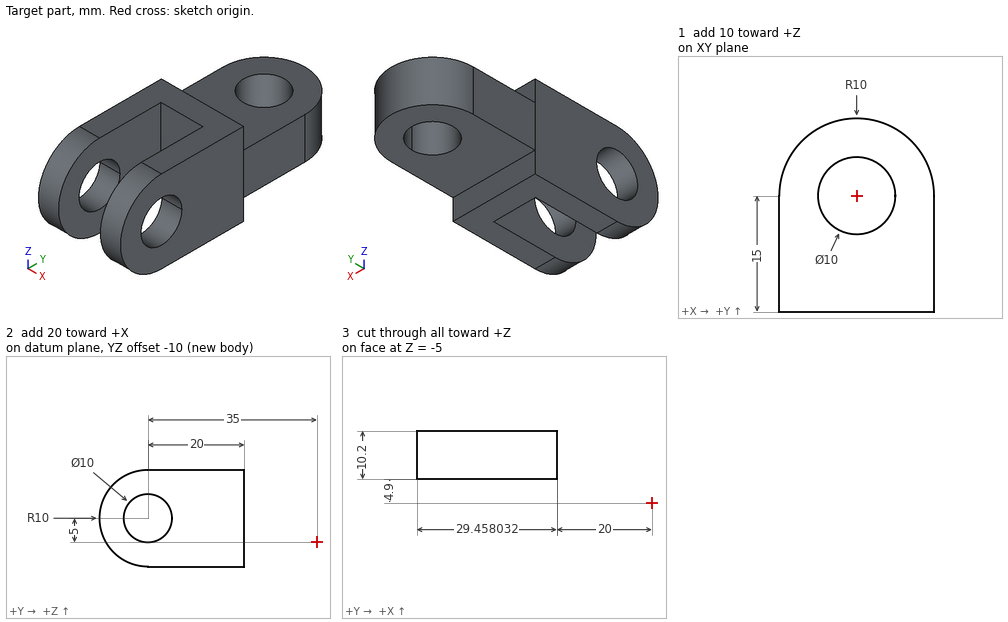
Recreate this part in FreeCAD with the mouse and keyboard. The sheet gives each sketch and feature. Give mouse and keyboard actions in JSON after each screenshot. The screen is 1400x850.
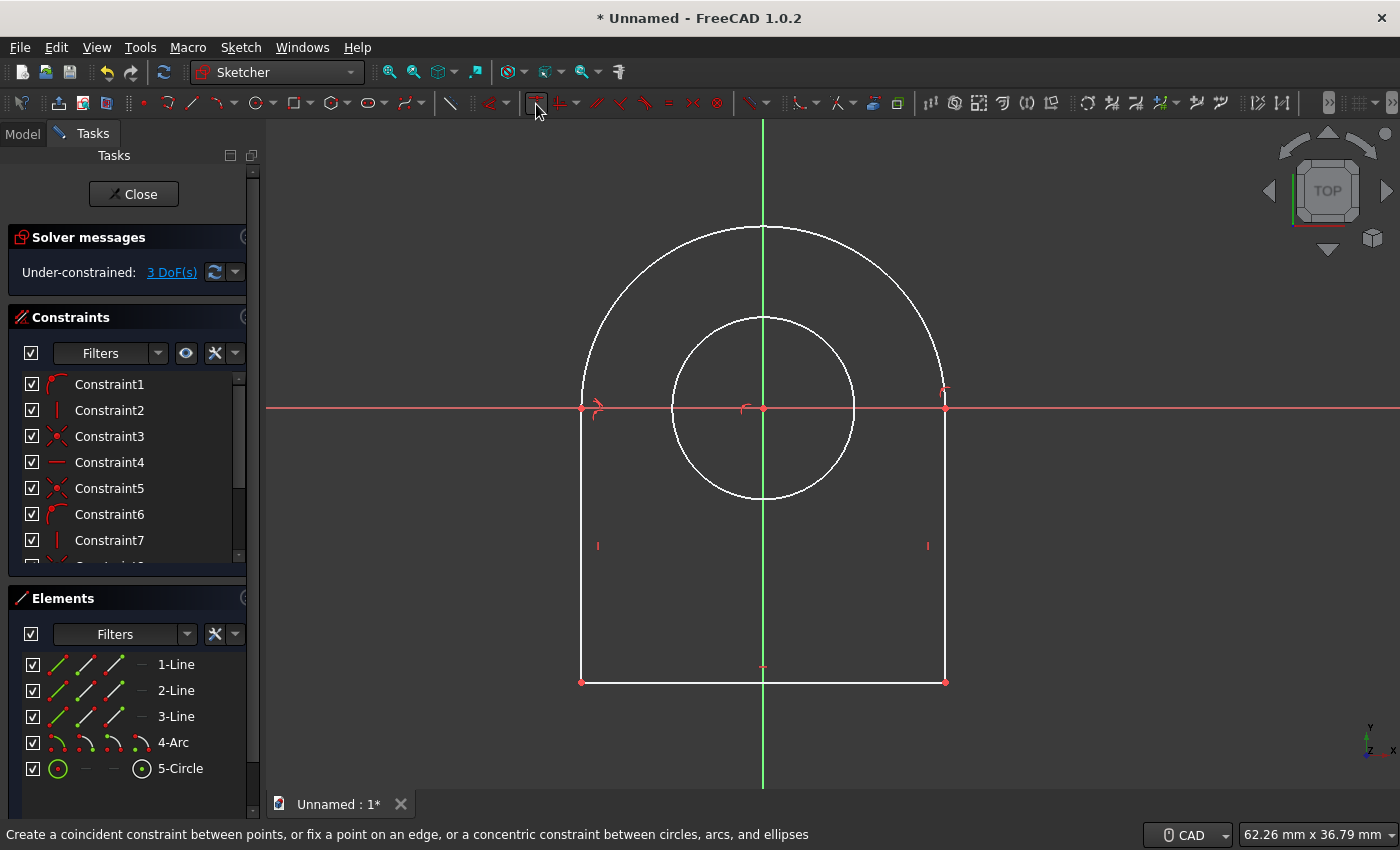
{"action": "left_click", "coordinate": [490, 104]}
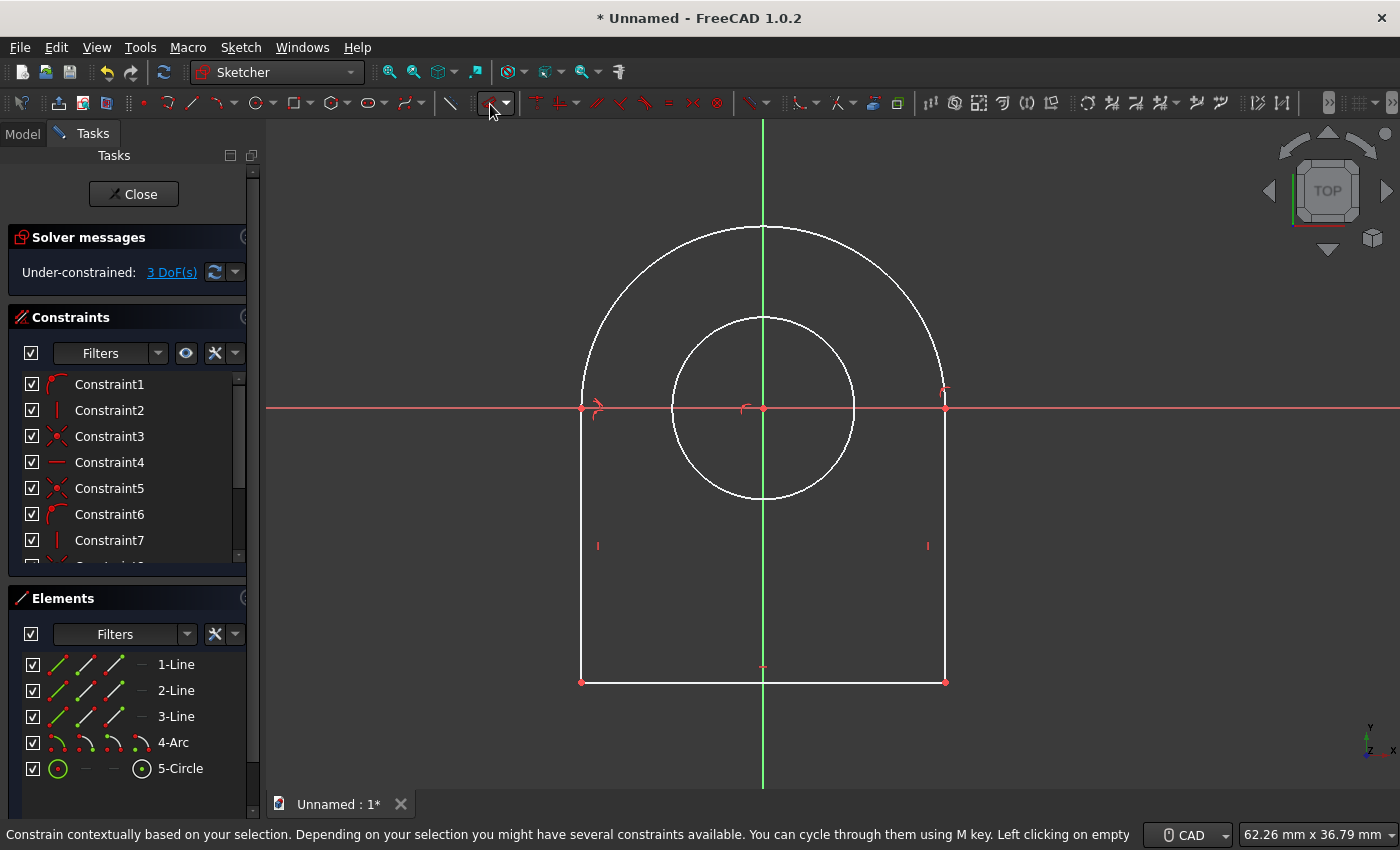
{"action": "left_click", "coordinate": [870, 261]}
{"action": "left_click", "coordinate": [889, 235]}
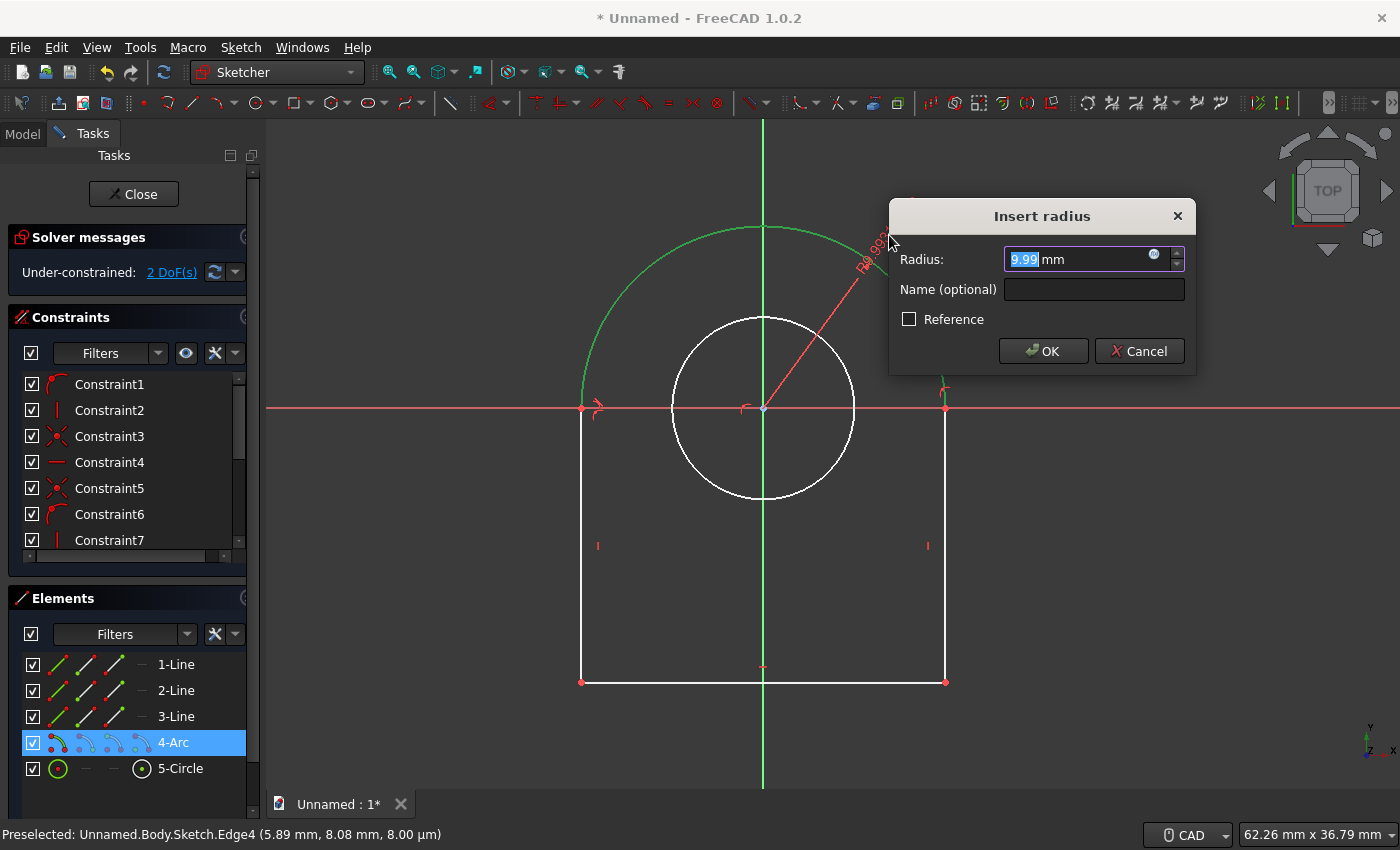
{"action": "type", "text": "10"}
{"action": "key", "text": "Return"}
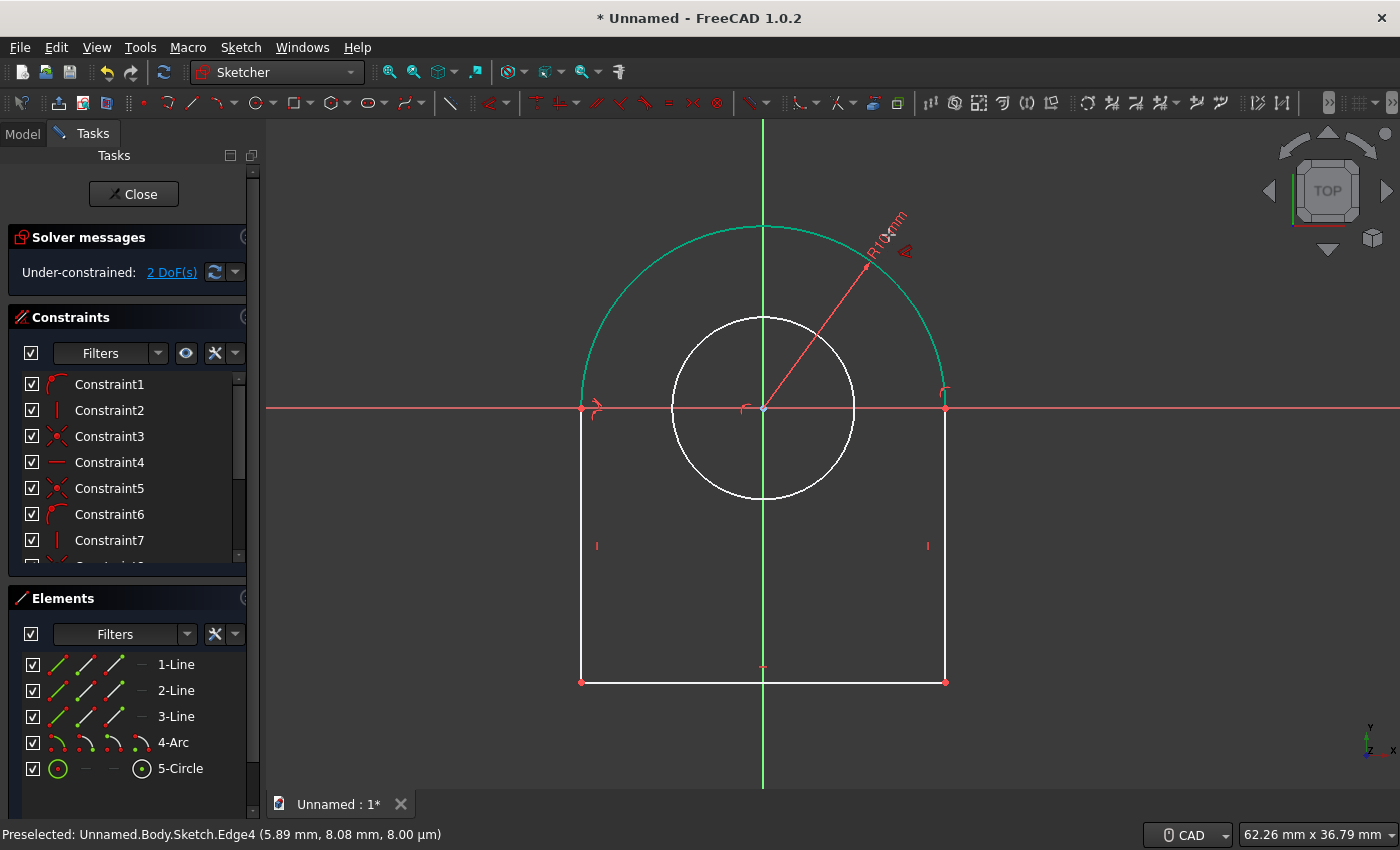
{"action": "left_click", "coordinate": [828, 344]}
{"action": "left_click", "coordinate": [851, 321]}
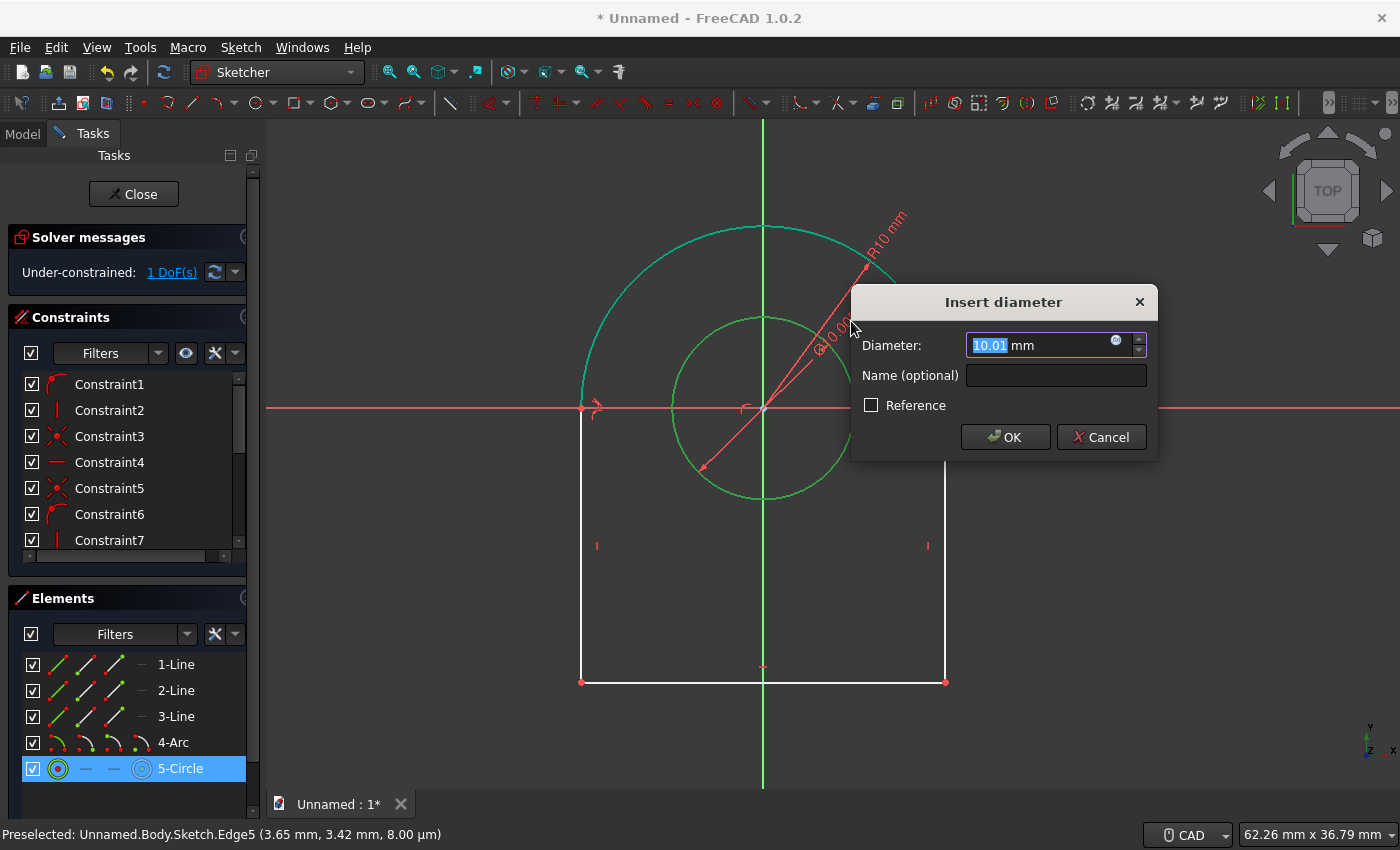
{"action": "type", "text": "10"}
{"action": "key", "text": "Return"}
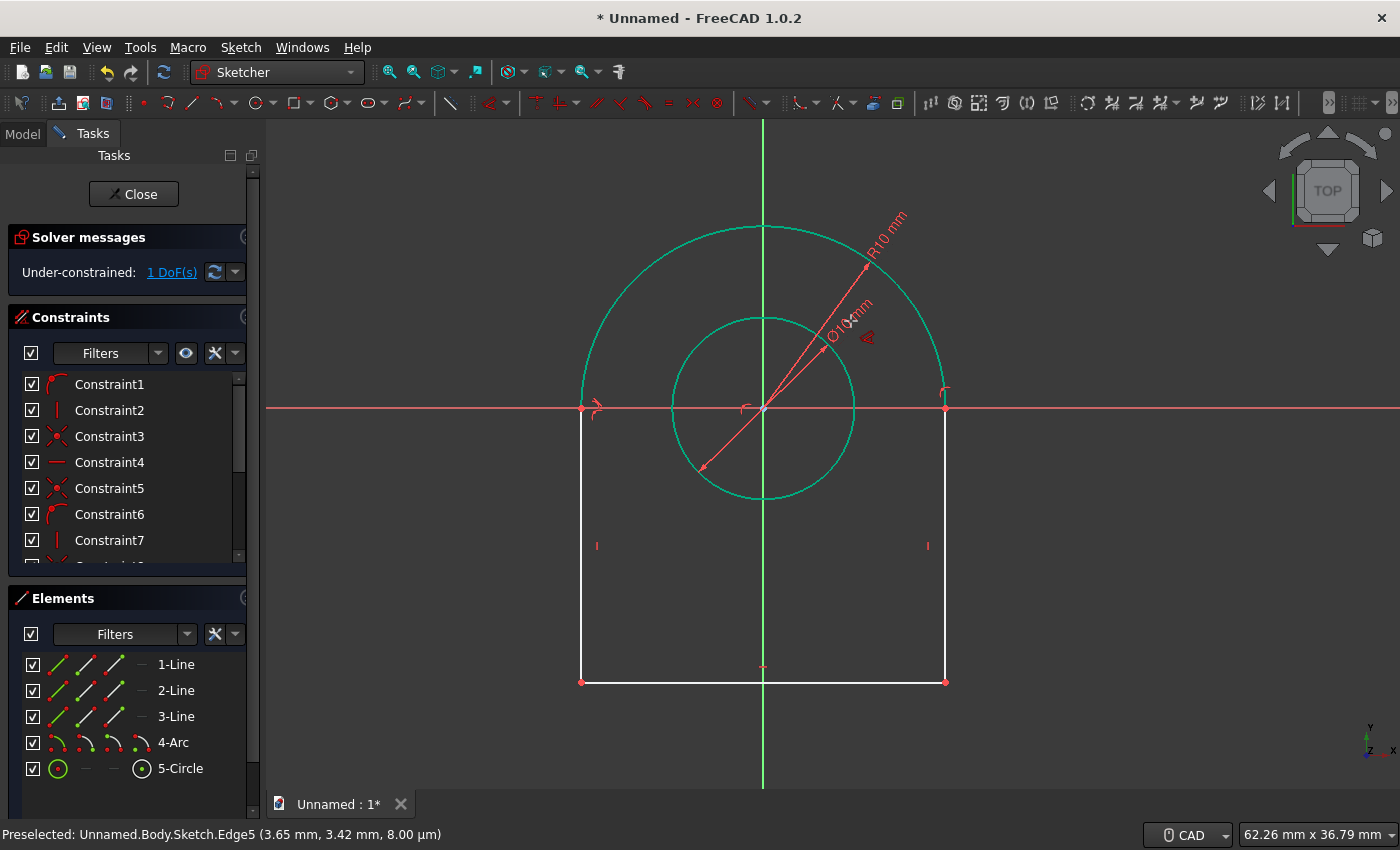
{"action": "left_click", "coordinate": [581, 491]}
{"action": "left_click", "coordinate": [547, 546]}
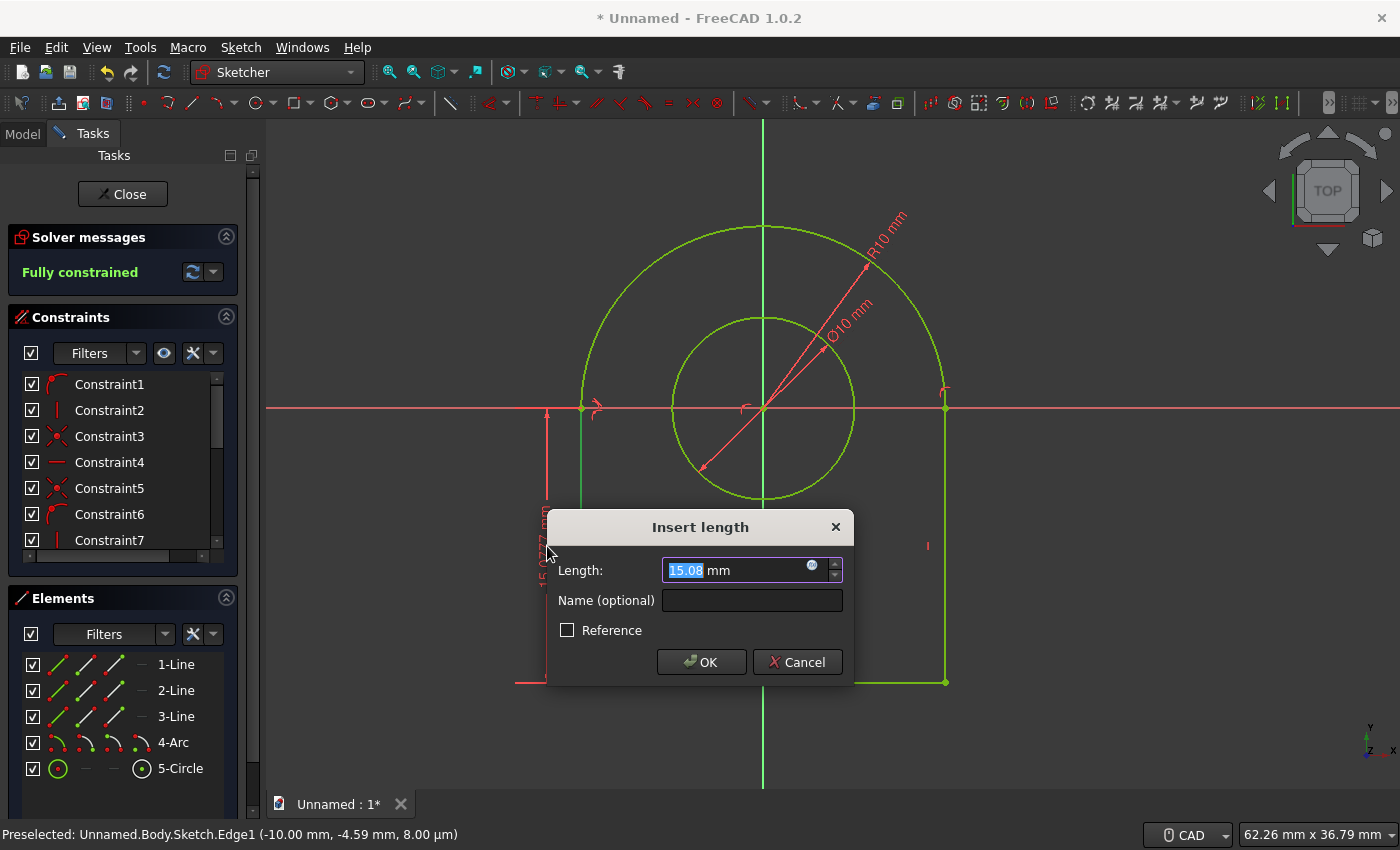
{"action": "type", "text": "15"}
{"action": "key", "text": "Return"}
{"action": "key", "text": "Escape"}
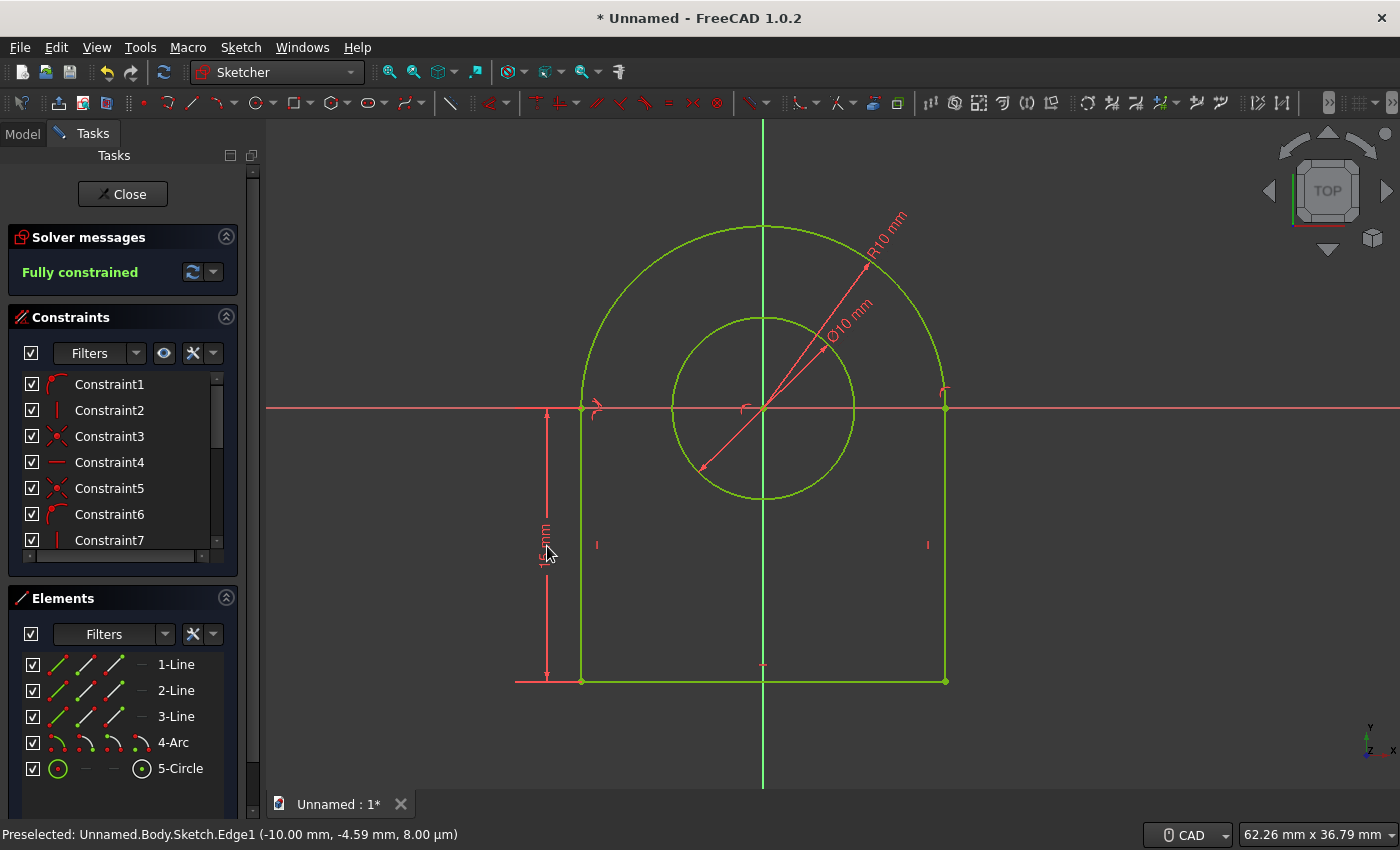
{"action": "left_click", "coordinate": [123, 194]}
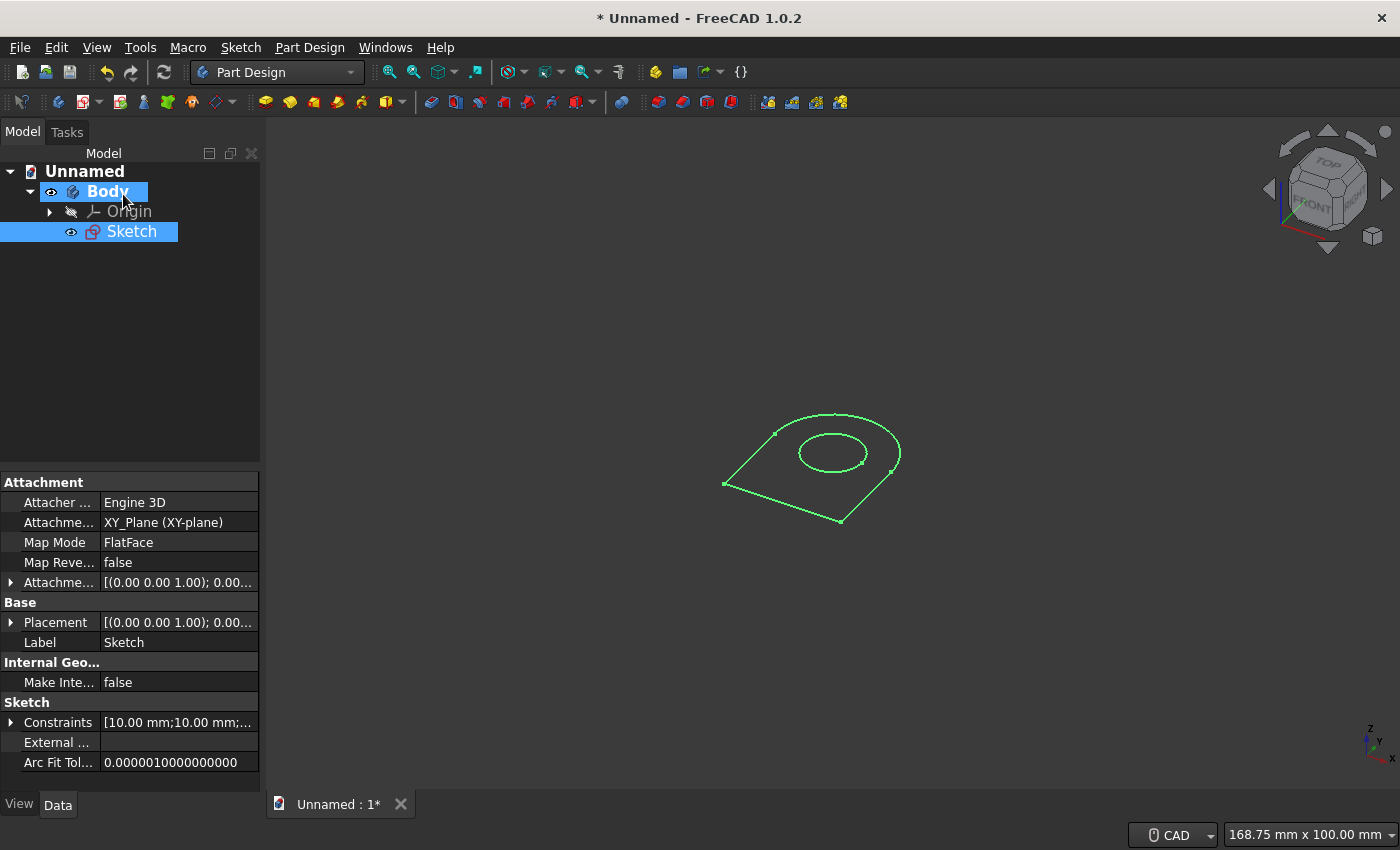
{"action": "left_click", "coordinate": [266, 102]}